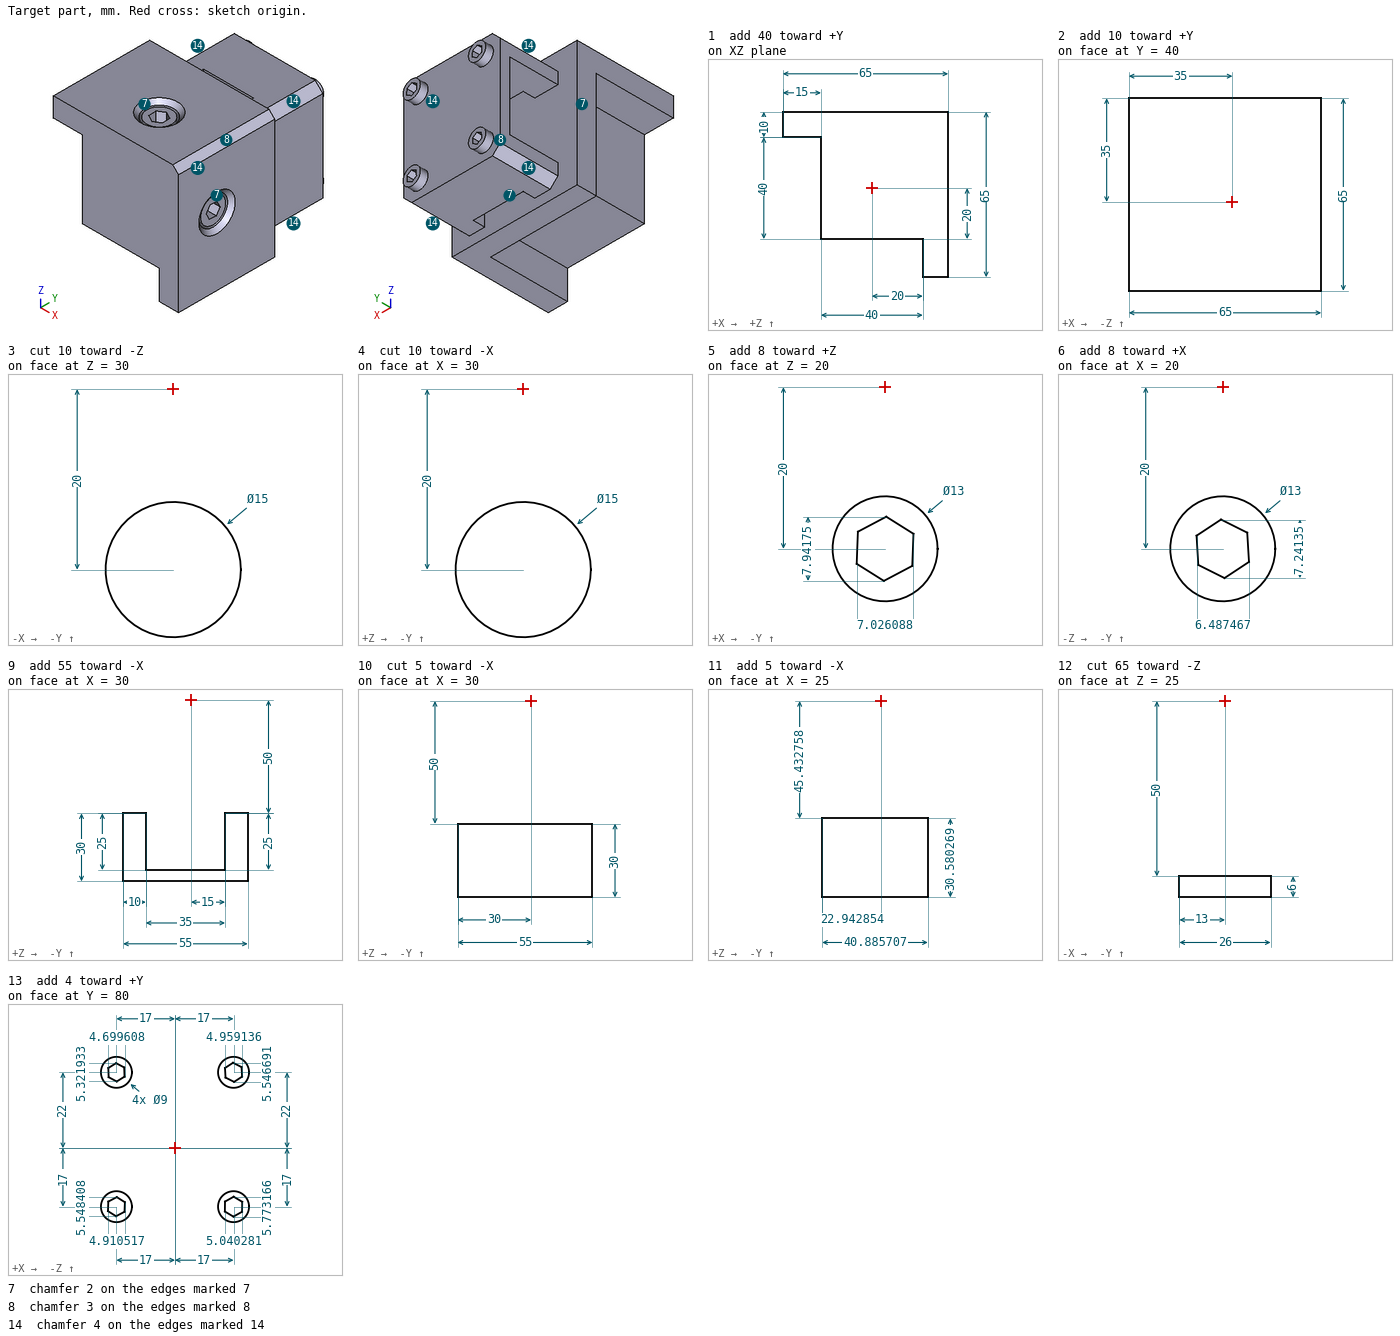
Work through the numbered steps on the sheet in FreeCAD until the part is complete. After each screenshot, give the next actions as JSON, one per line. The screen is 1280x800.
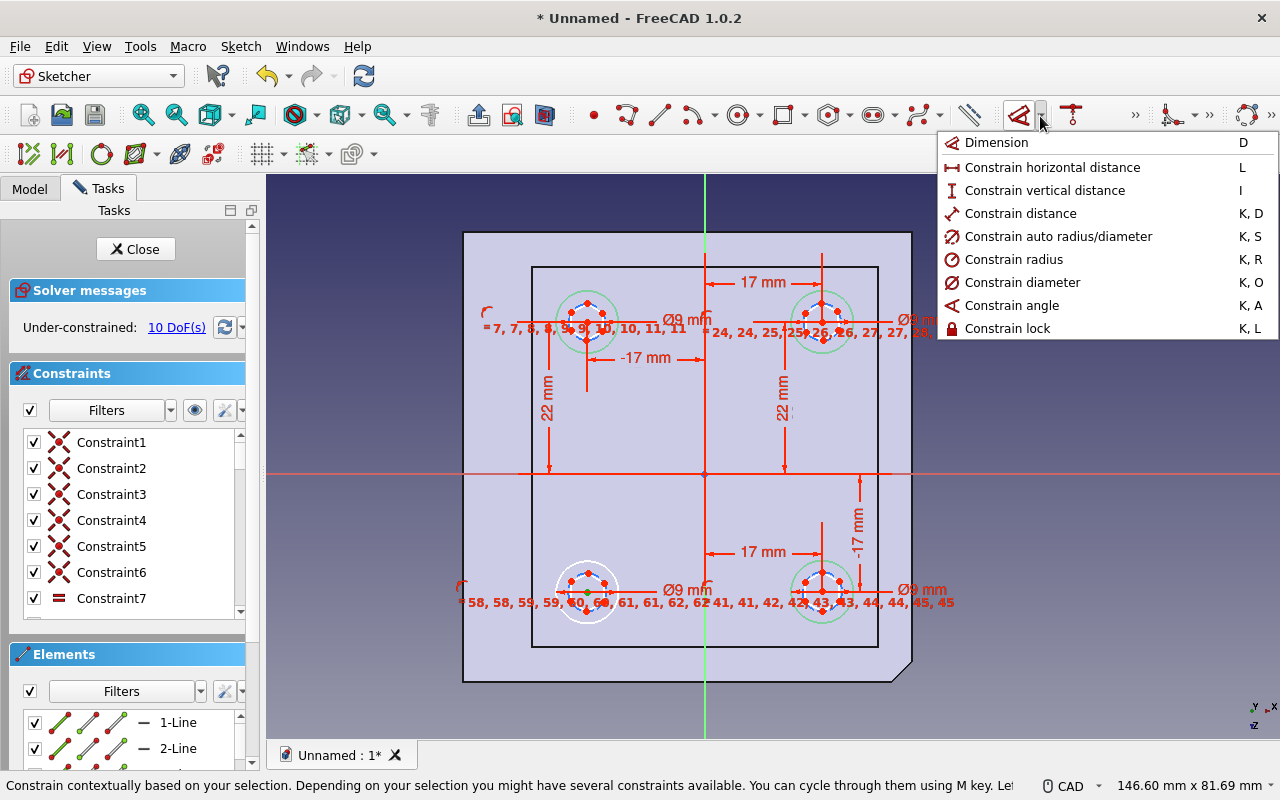
{"action": "left_click", "coordinate": [1108, 168]}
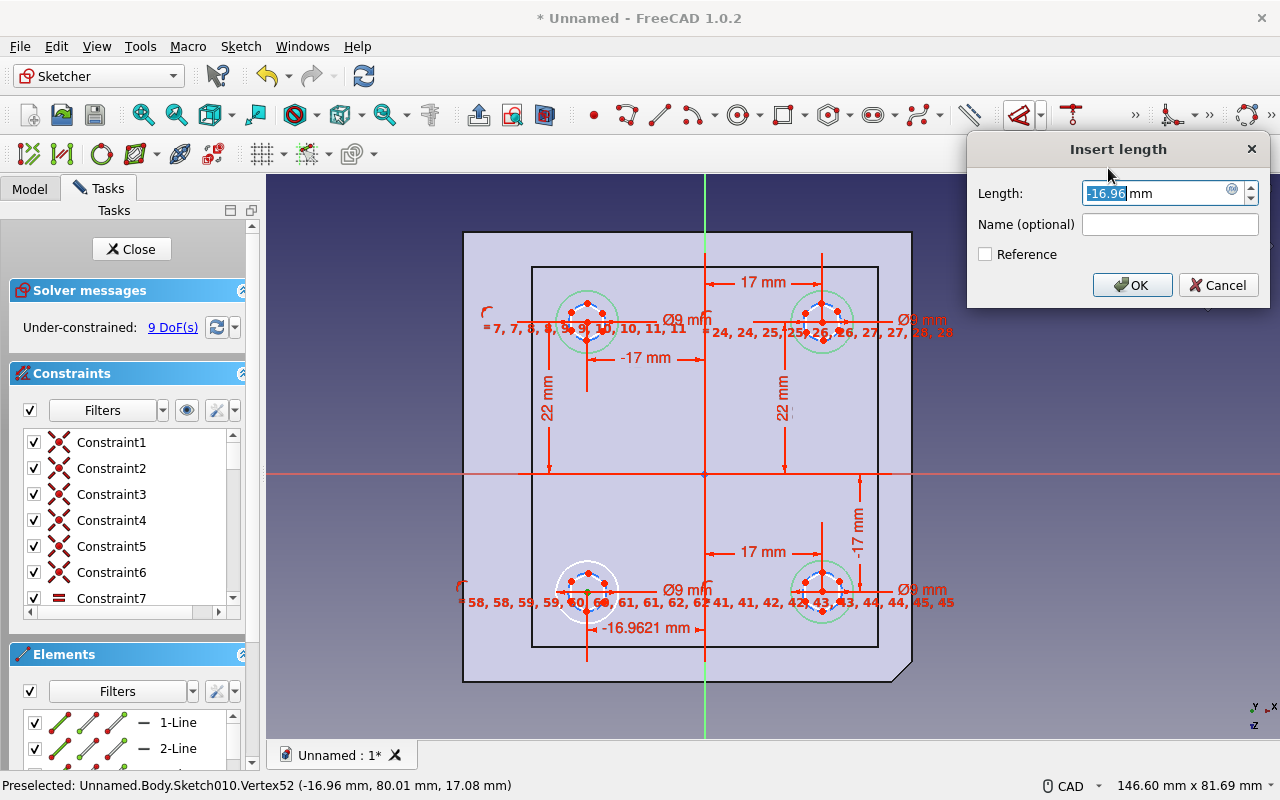
{"action": "type", "text": "-17"}
{"action": "key", "text": "Return"}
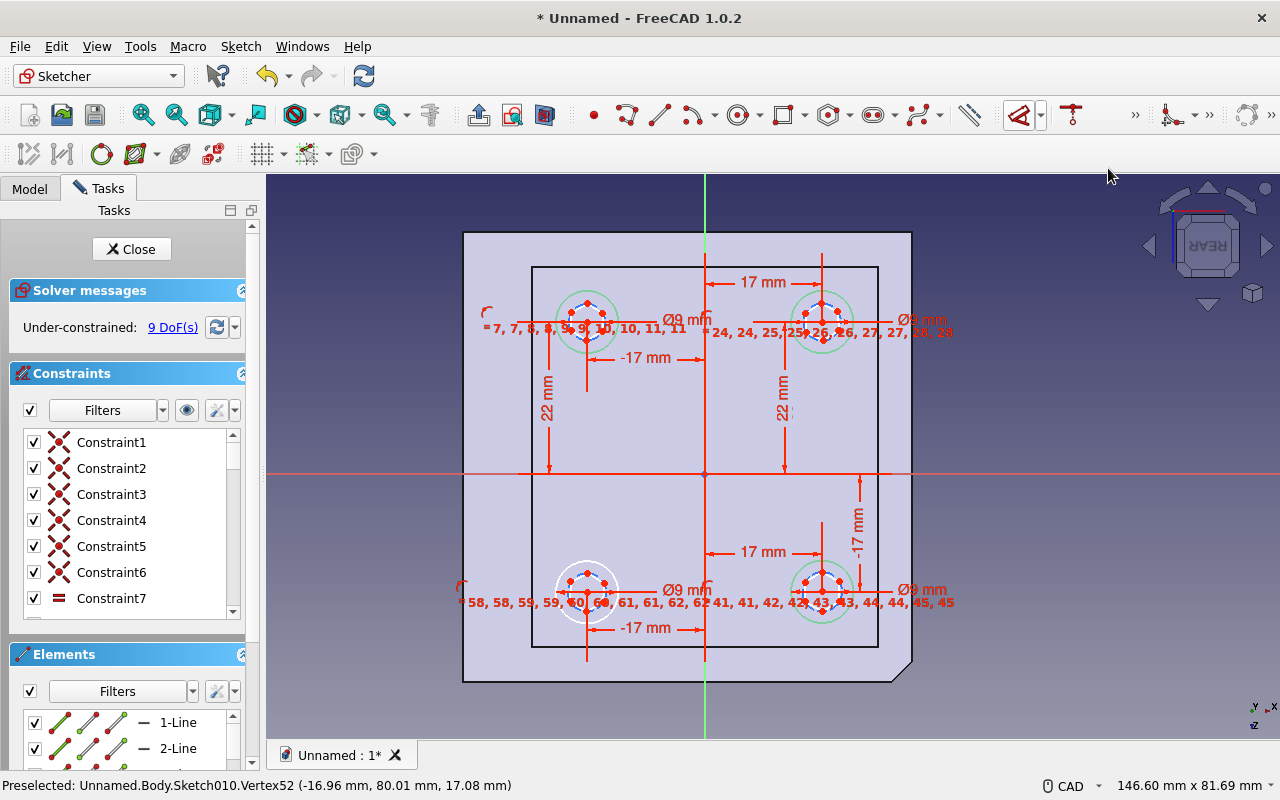
{"action": "left_click", "coordinate": [587, 592]}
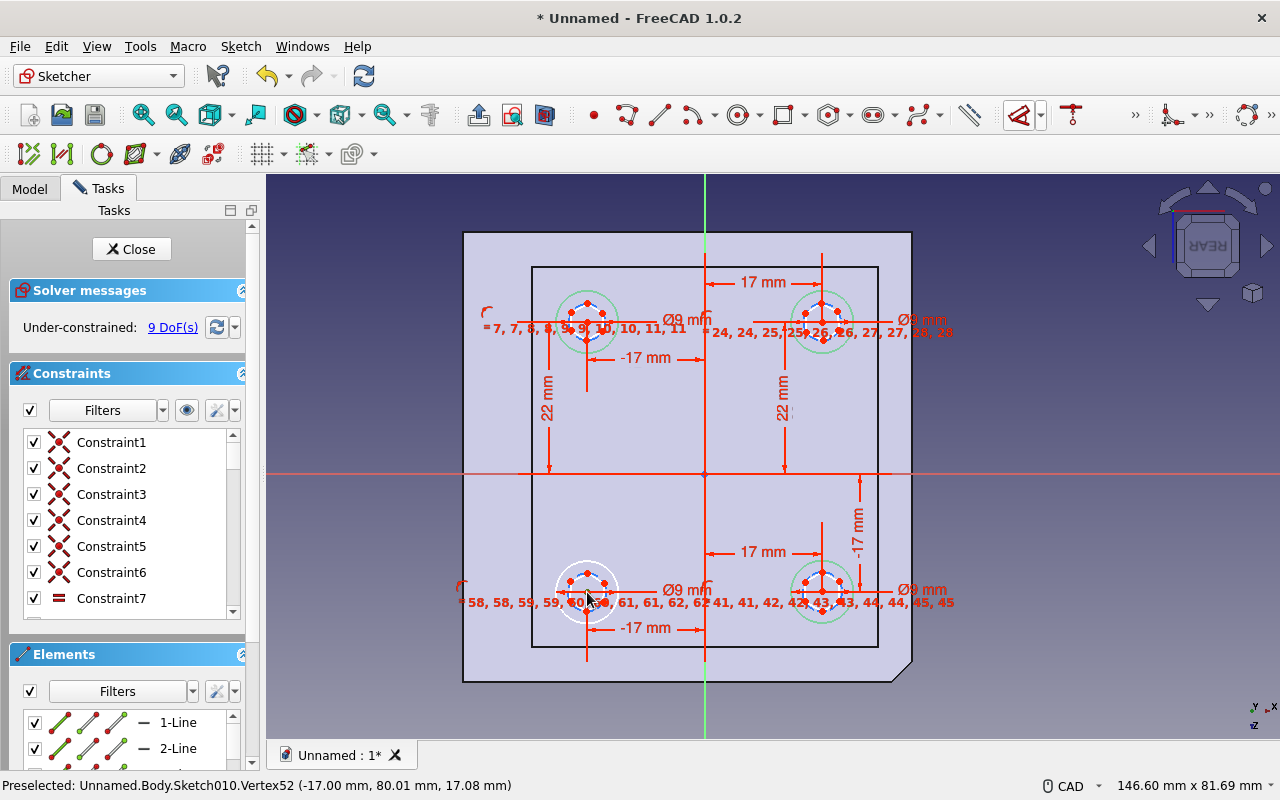
{"action": "key", "text": "i"}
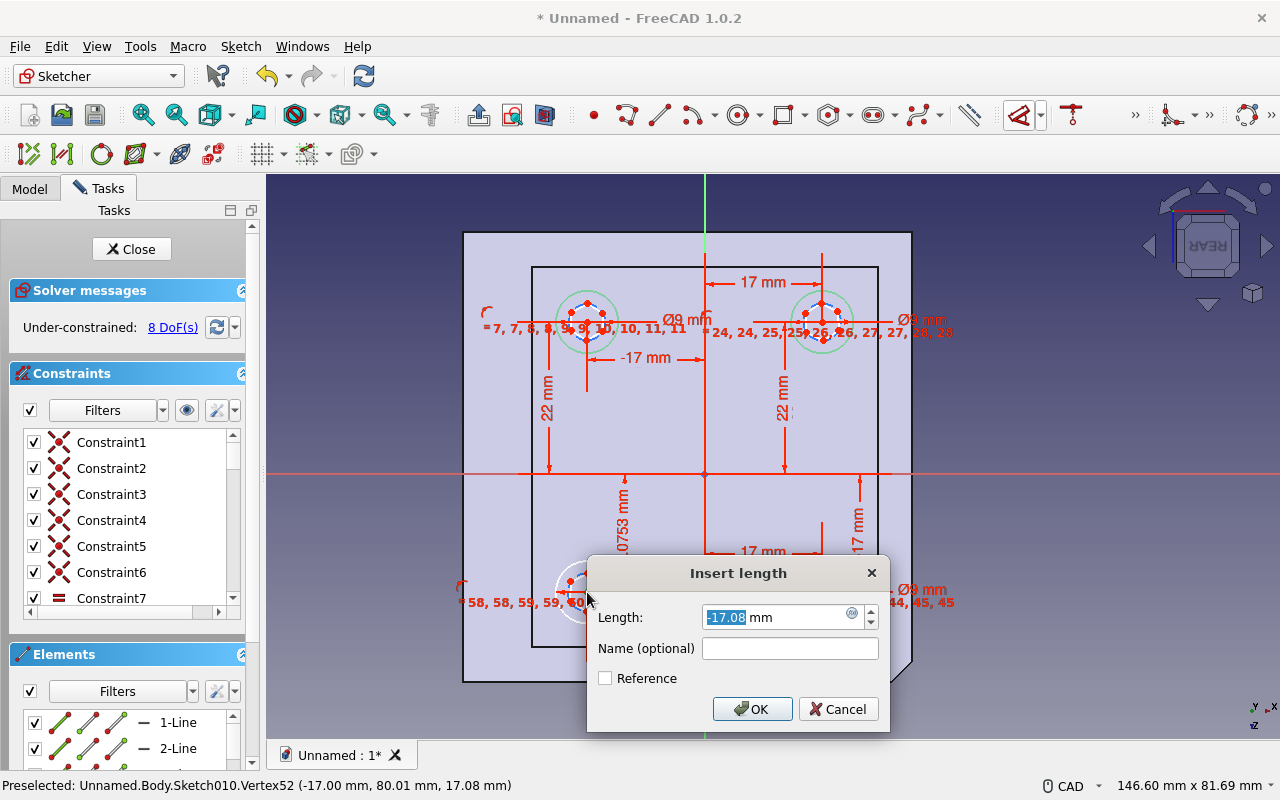
{"action": "type", "text": "-17"}
{"action": "key", "text": "Return"}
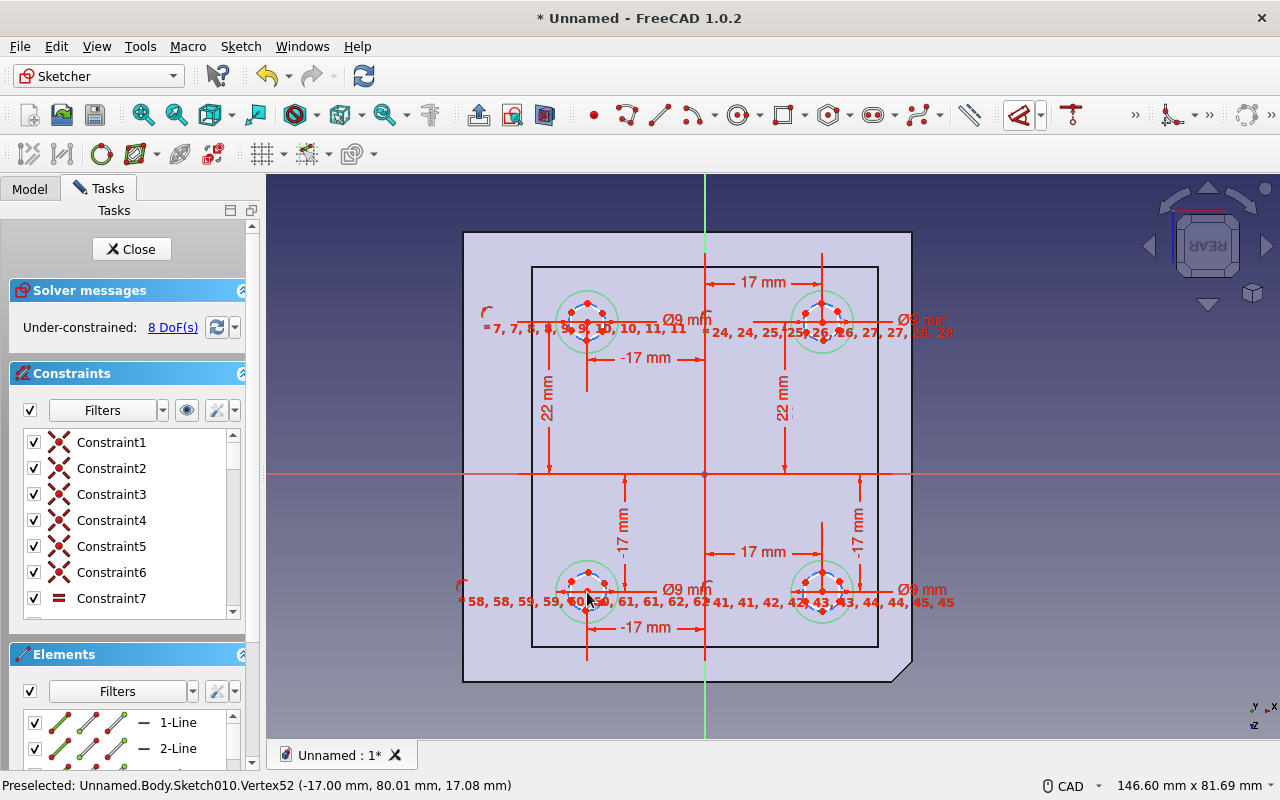
{"action": "left_click", "coordinate": [571, 313]}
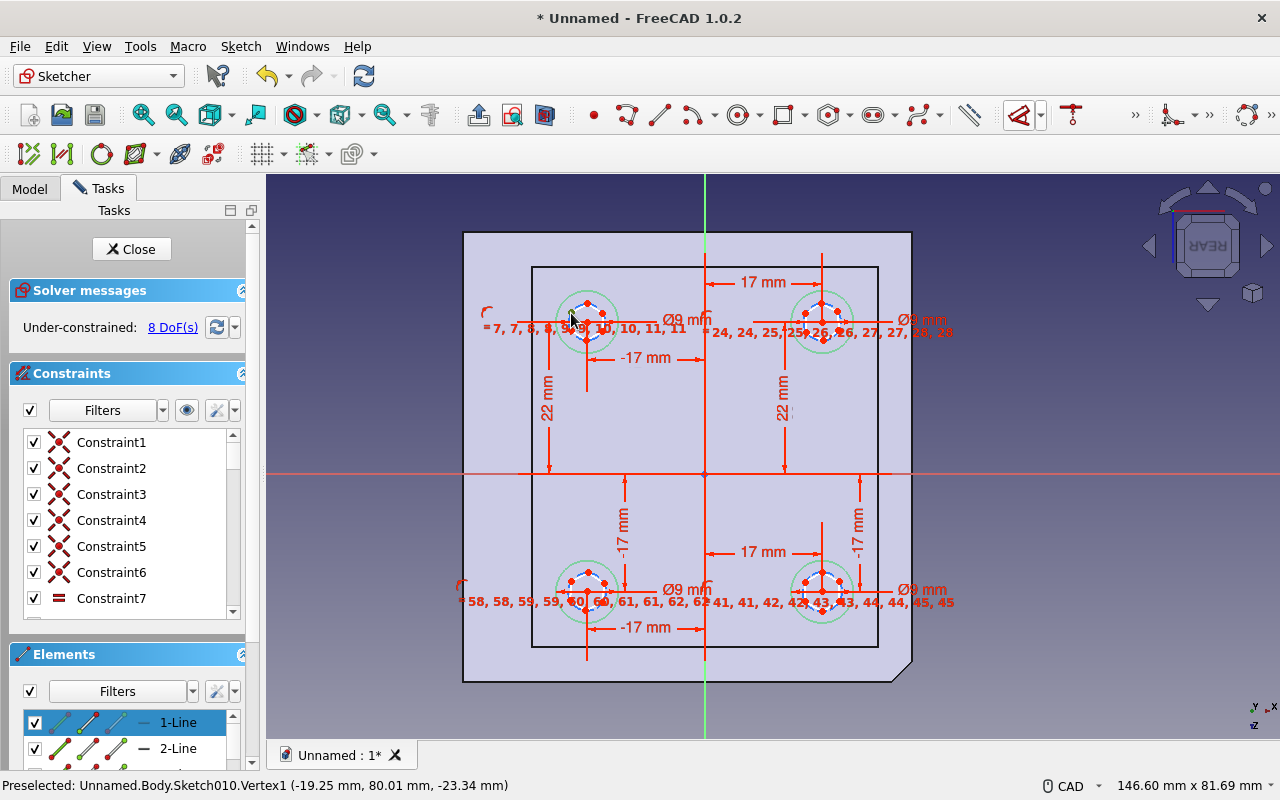
{"action": "left_click", "coordinate": [603, 331]}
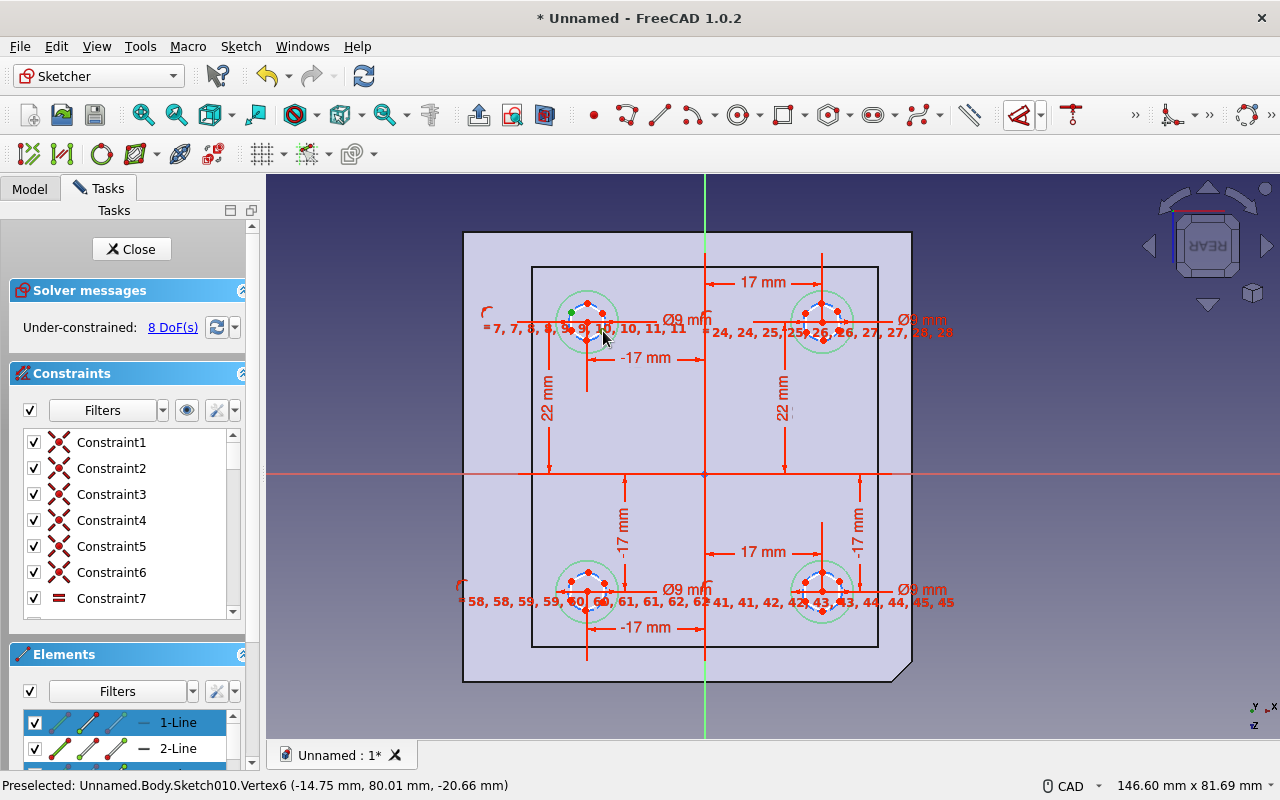
{"action": "key", "text": "l"}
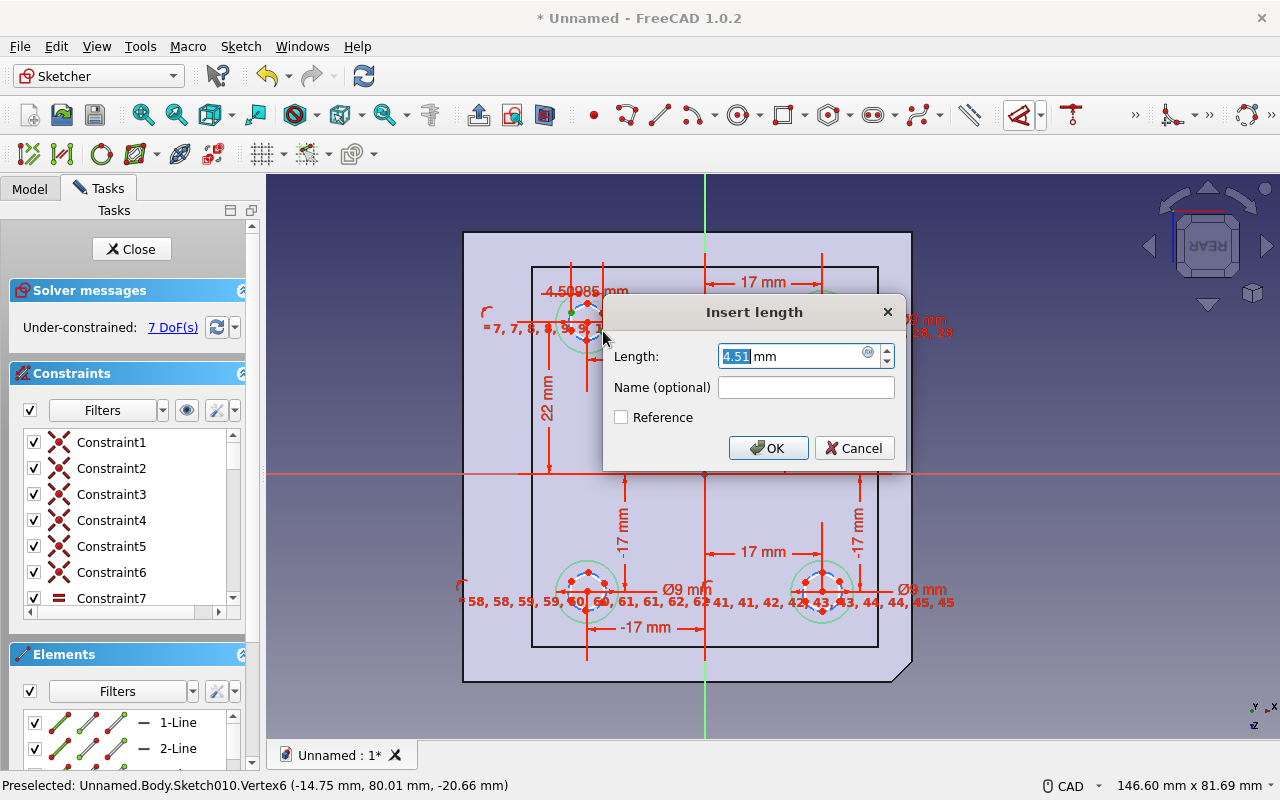
{"action": "type", "text": "4.699608"}
{"action": "key", "text": "Return"}